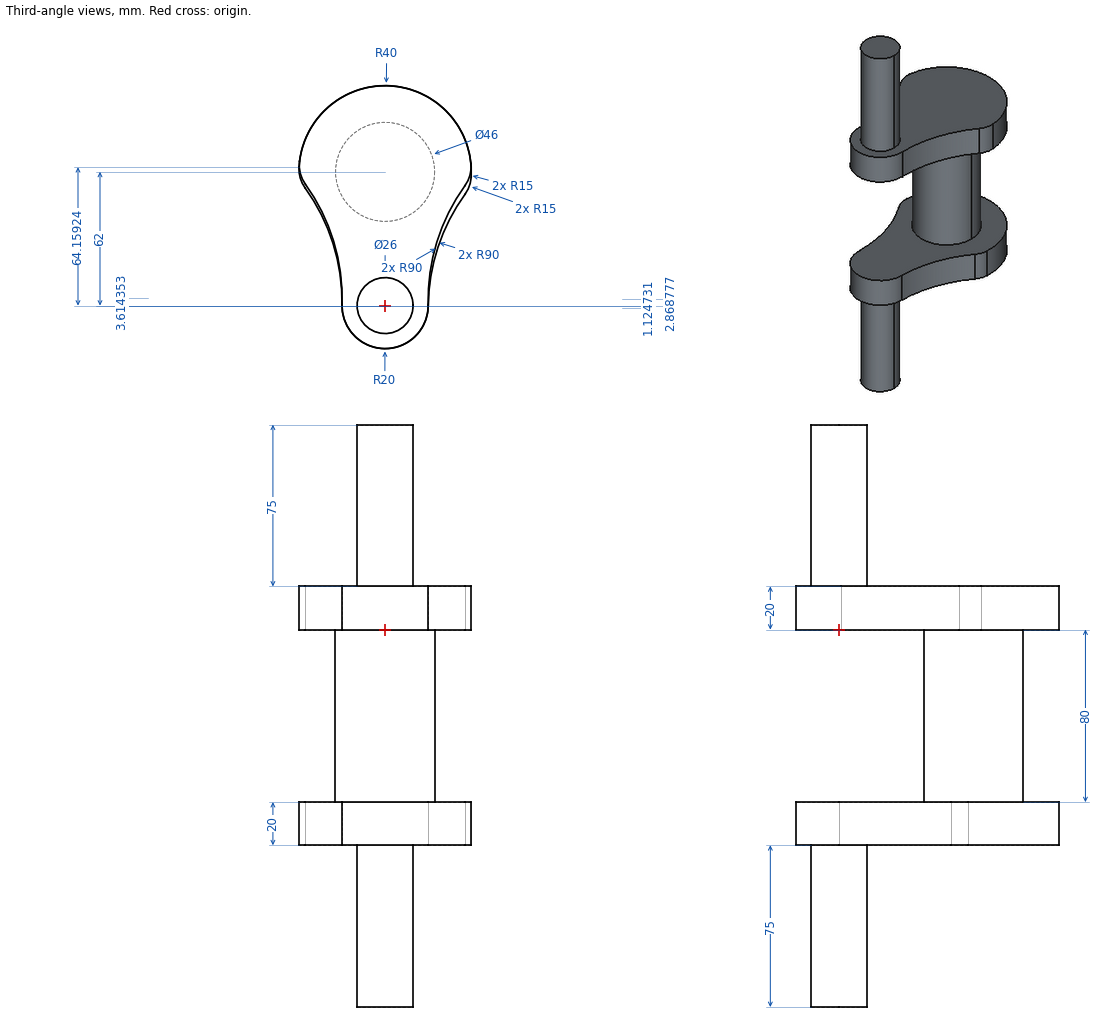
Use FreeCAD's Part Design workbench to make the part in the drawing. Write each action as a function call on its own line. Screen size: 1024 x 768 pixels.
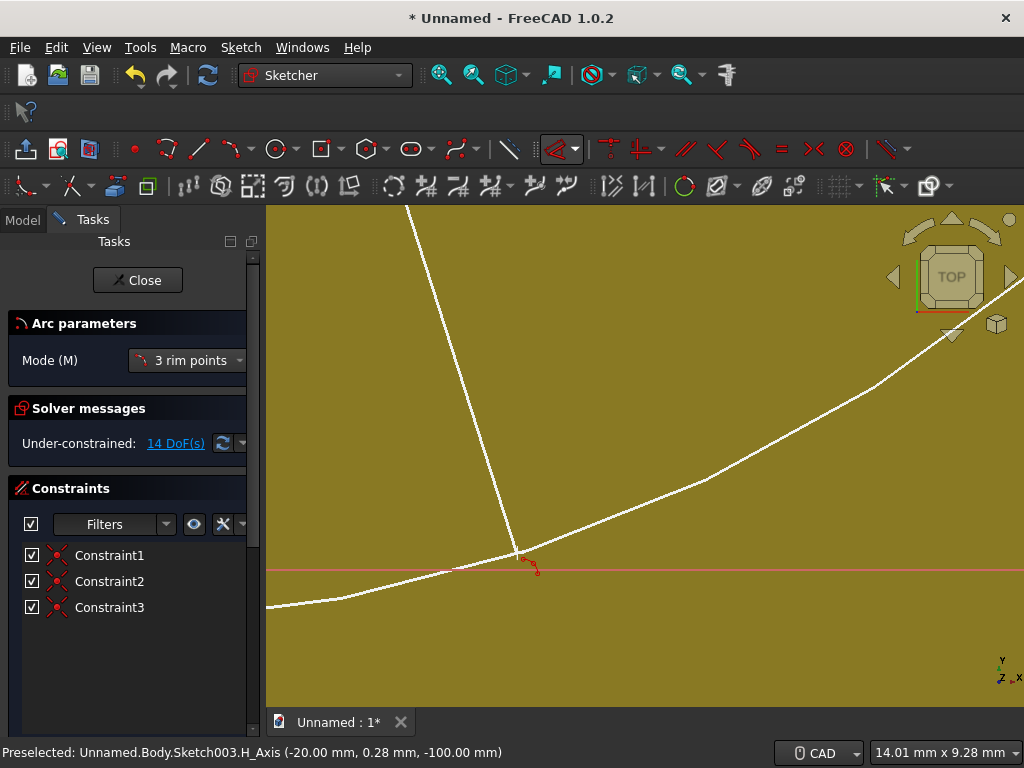
scroll(523, 566, down, 15)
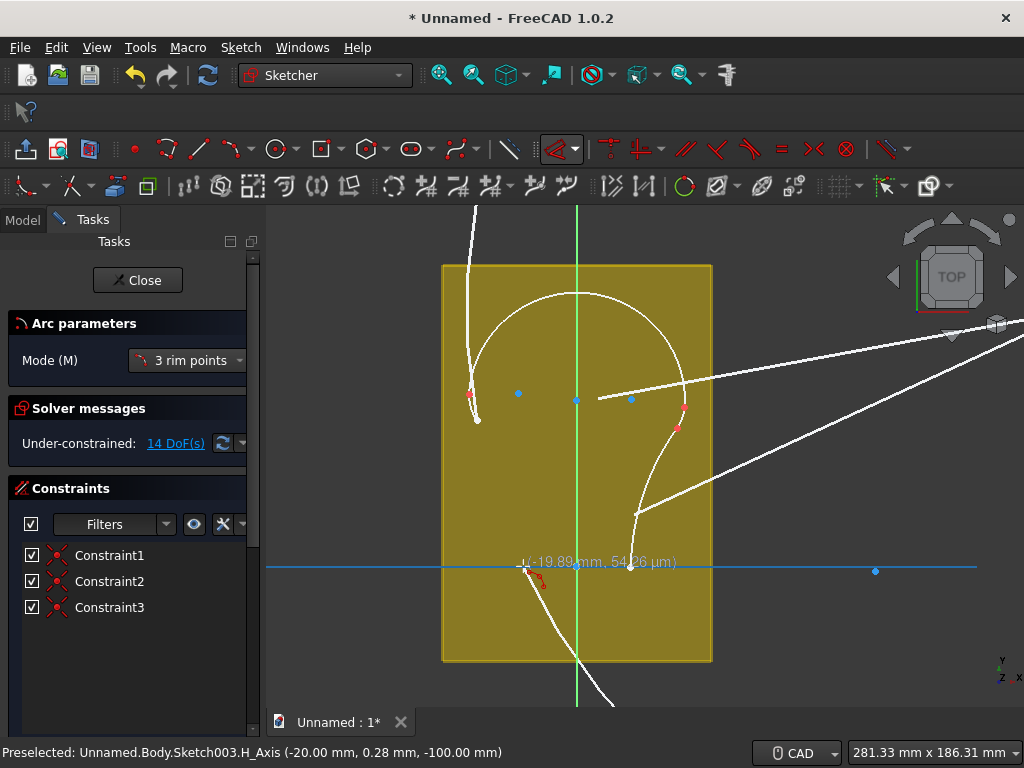
scroll(512, 489, up, 2)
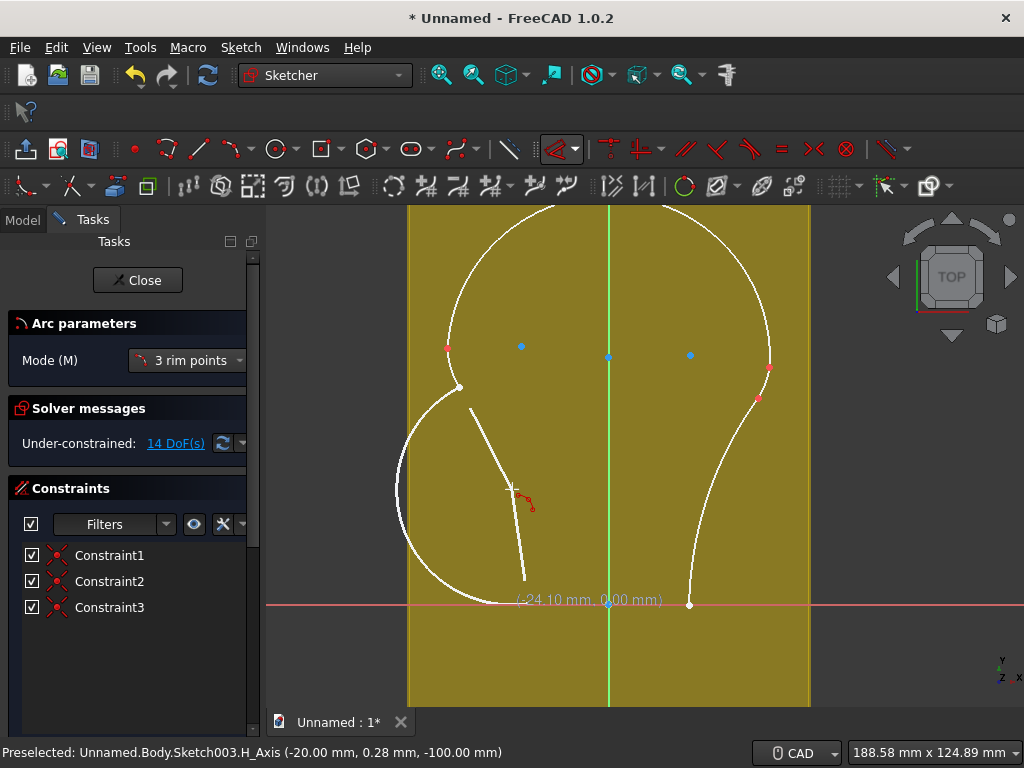
click(512, 489)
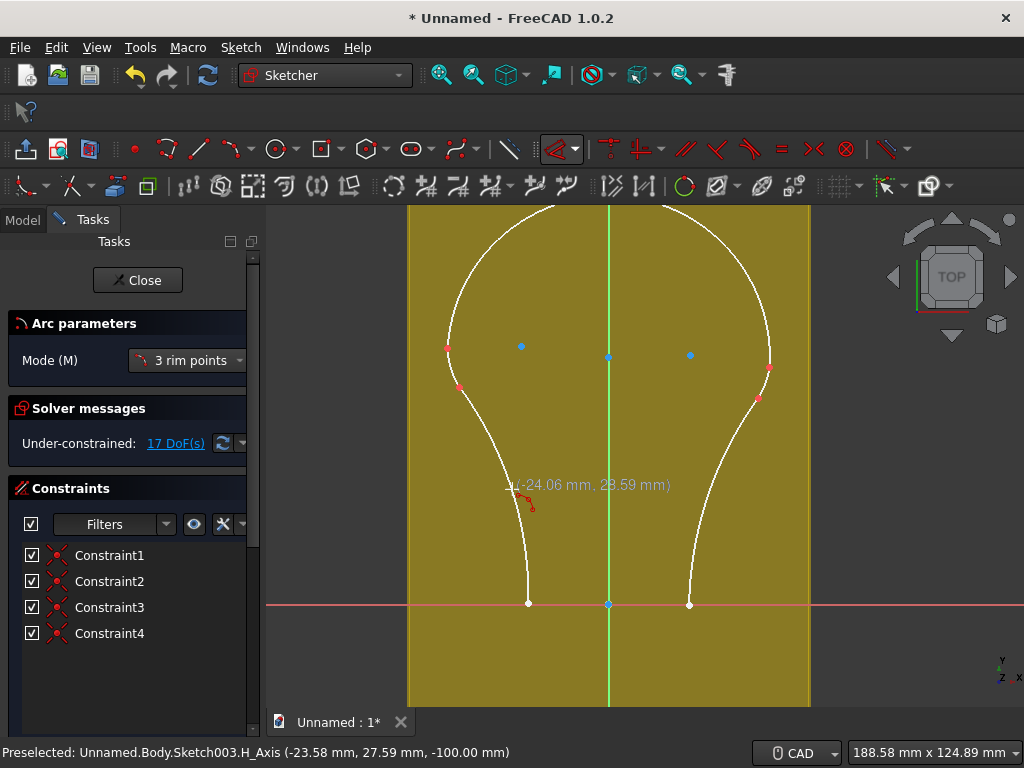
scroll(528, 604, up, 13)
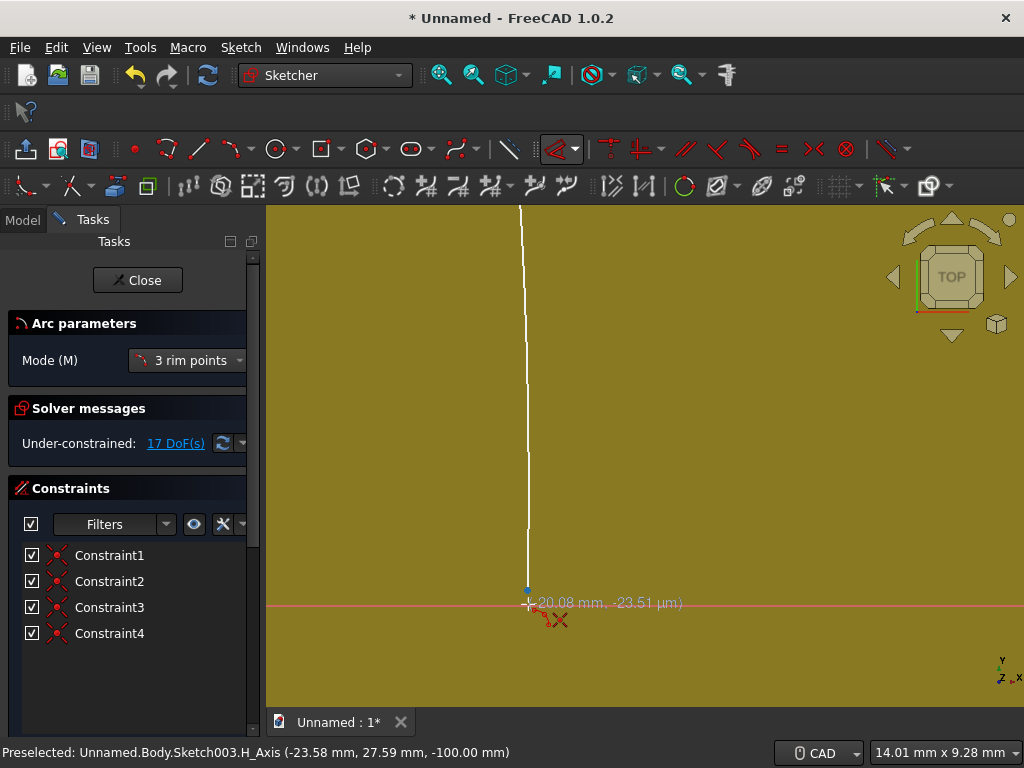
click(528, 590)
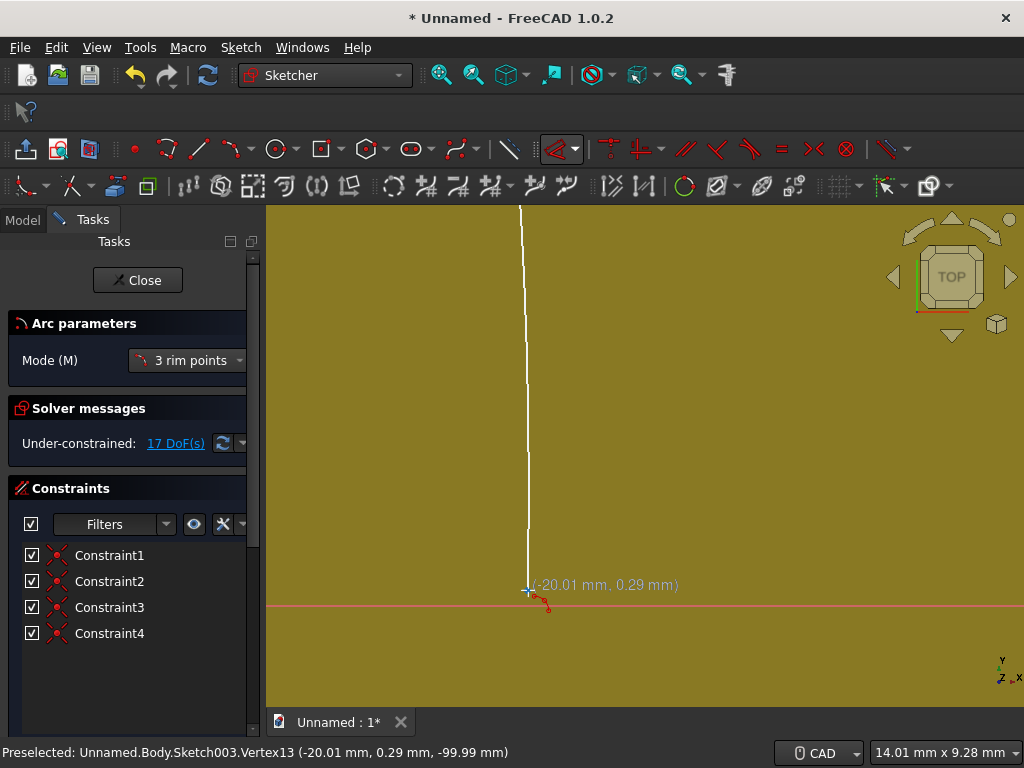
scroll(522, 564, down, 15)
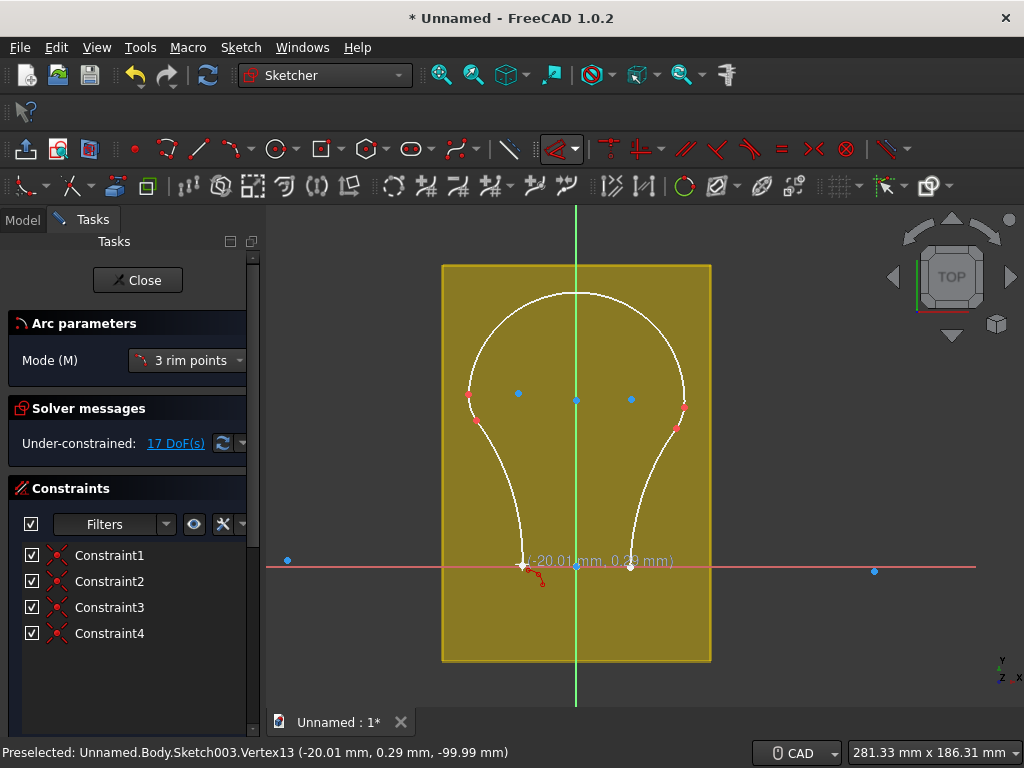
scroll(630, 567, up, 17)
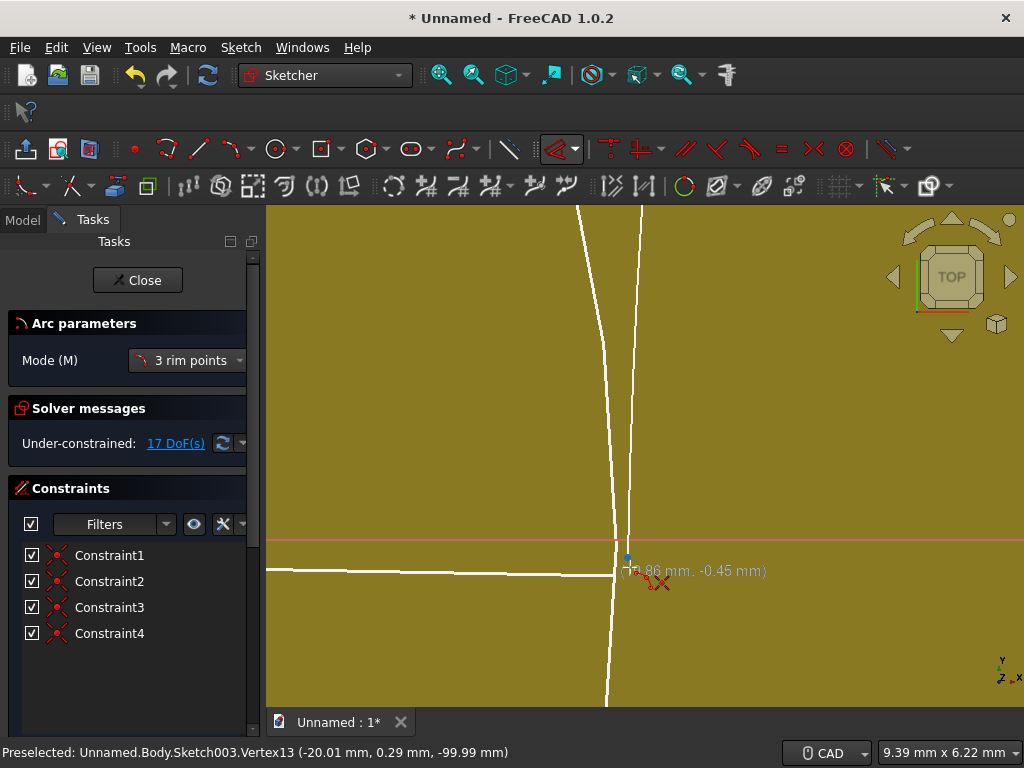
click(628, 557)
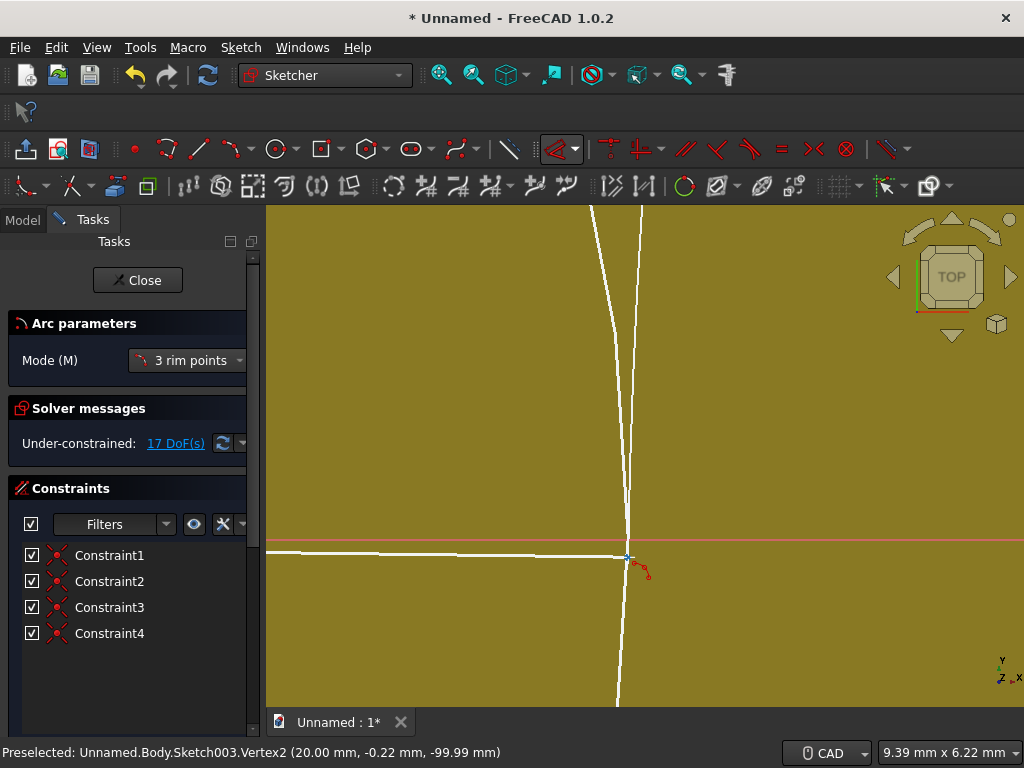
scroll(631, 567, down, 17)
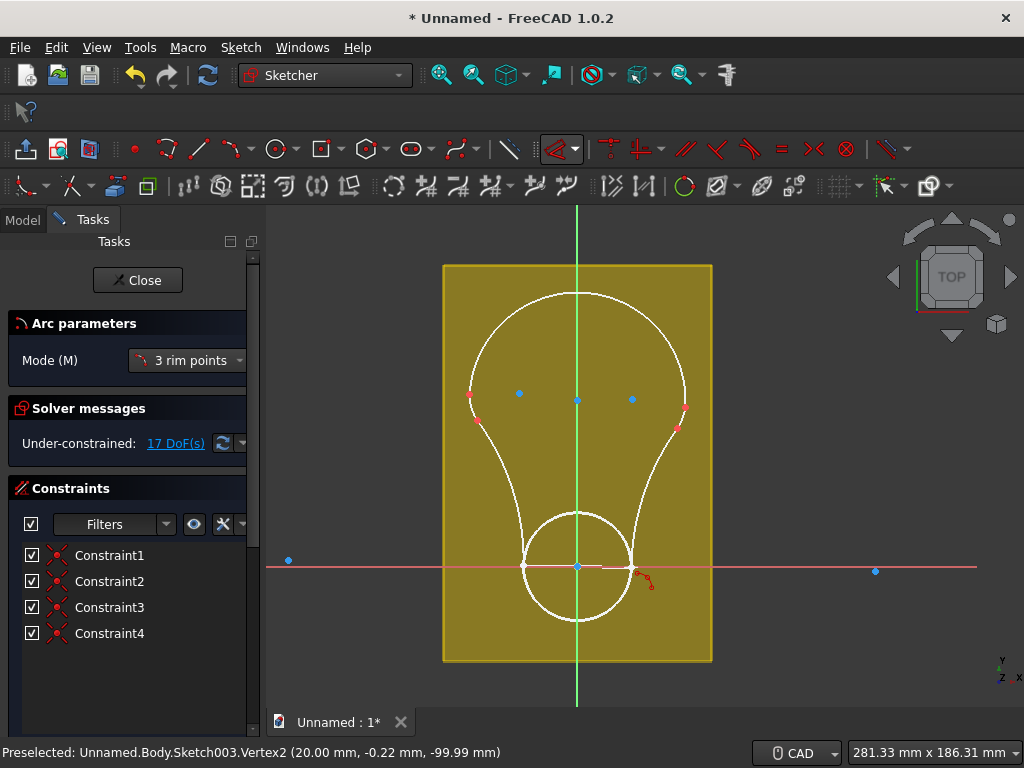
click(560, 618)
key(Escape)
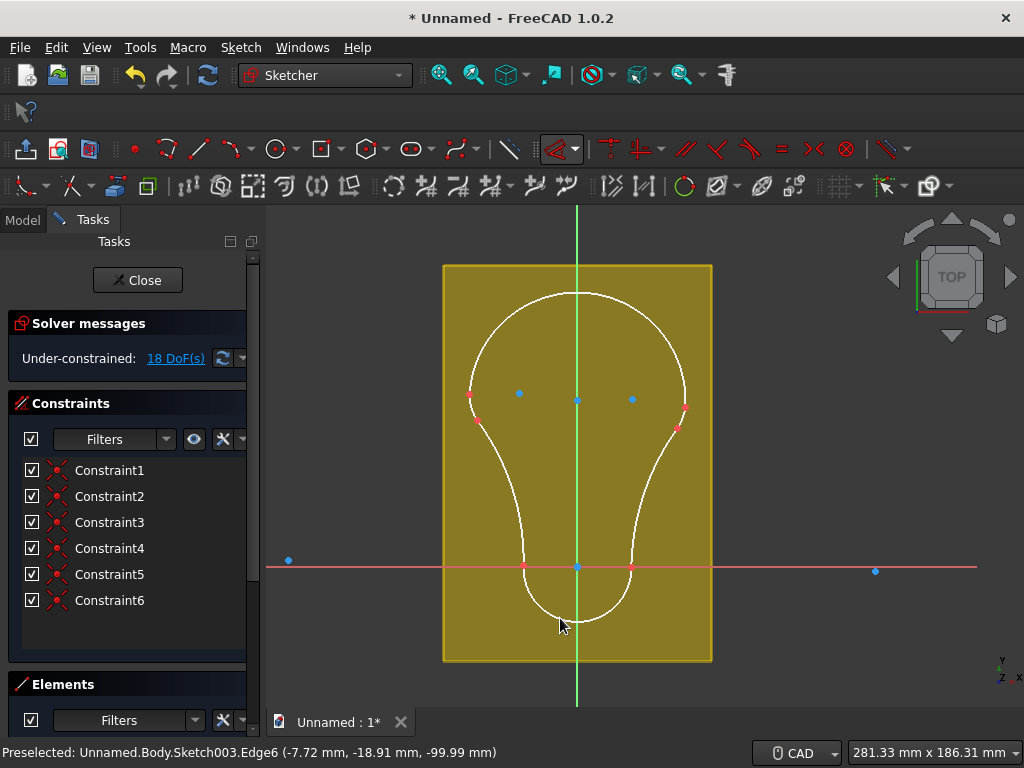
click(655, 467)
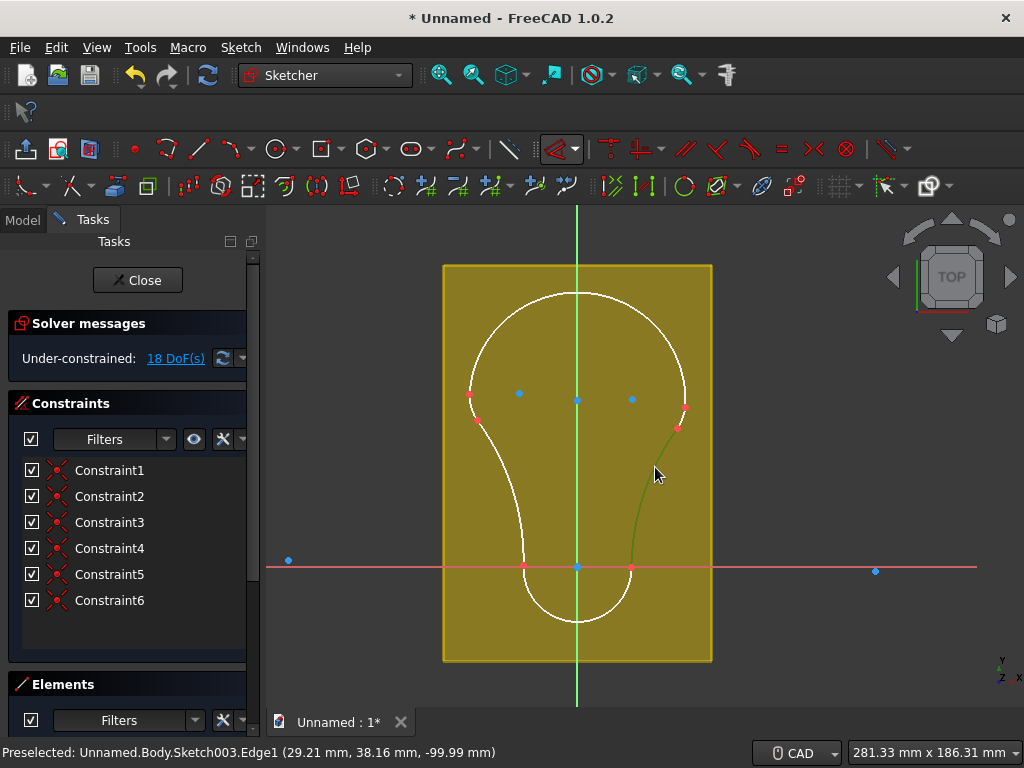
scroll(683, 418, up, 2)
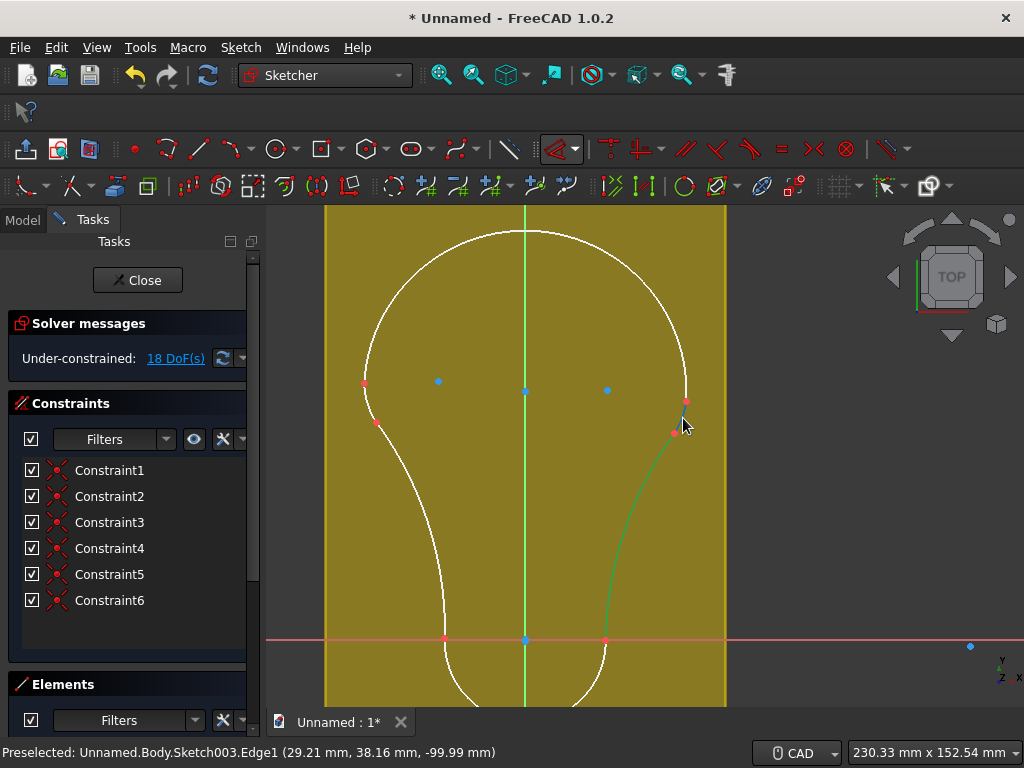
click(682, 418)